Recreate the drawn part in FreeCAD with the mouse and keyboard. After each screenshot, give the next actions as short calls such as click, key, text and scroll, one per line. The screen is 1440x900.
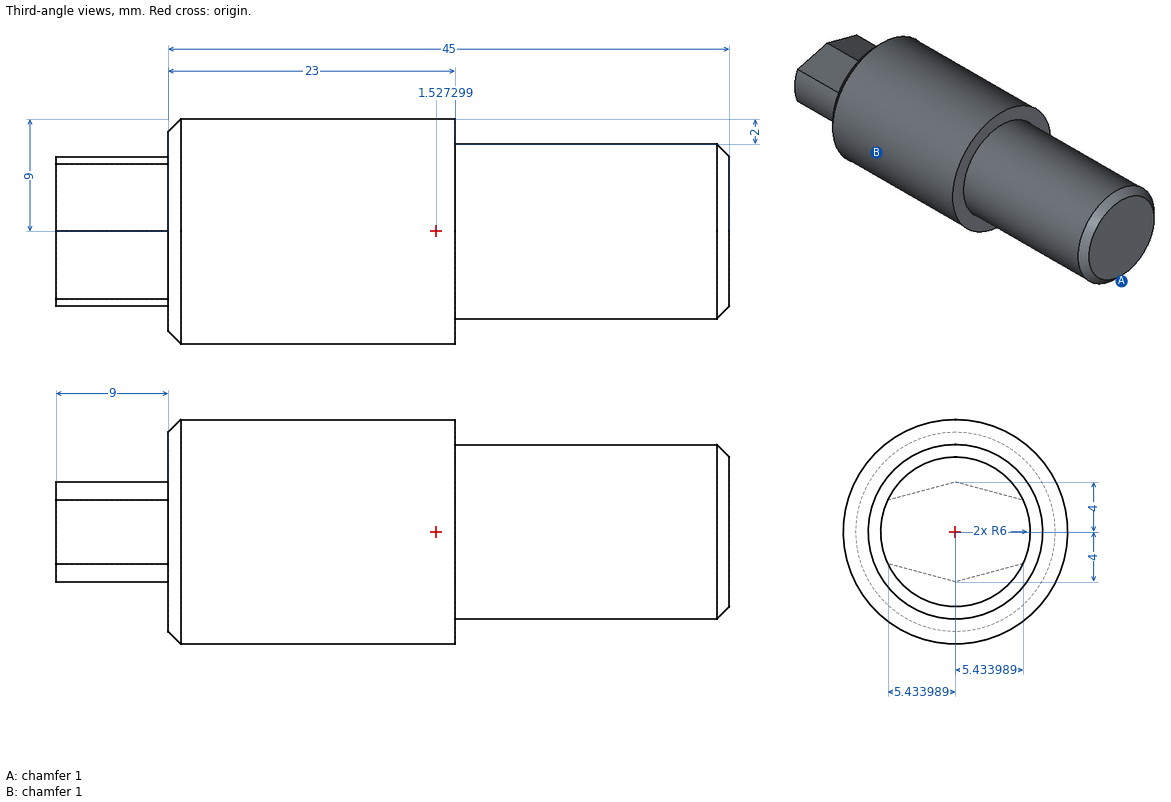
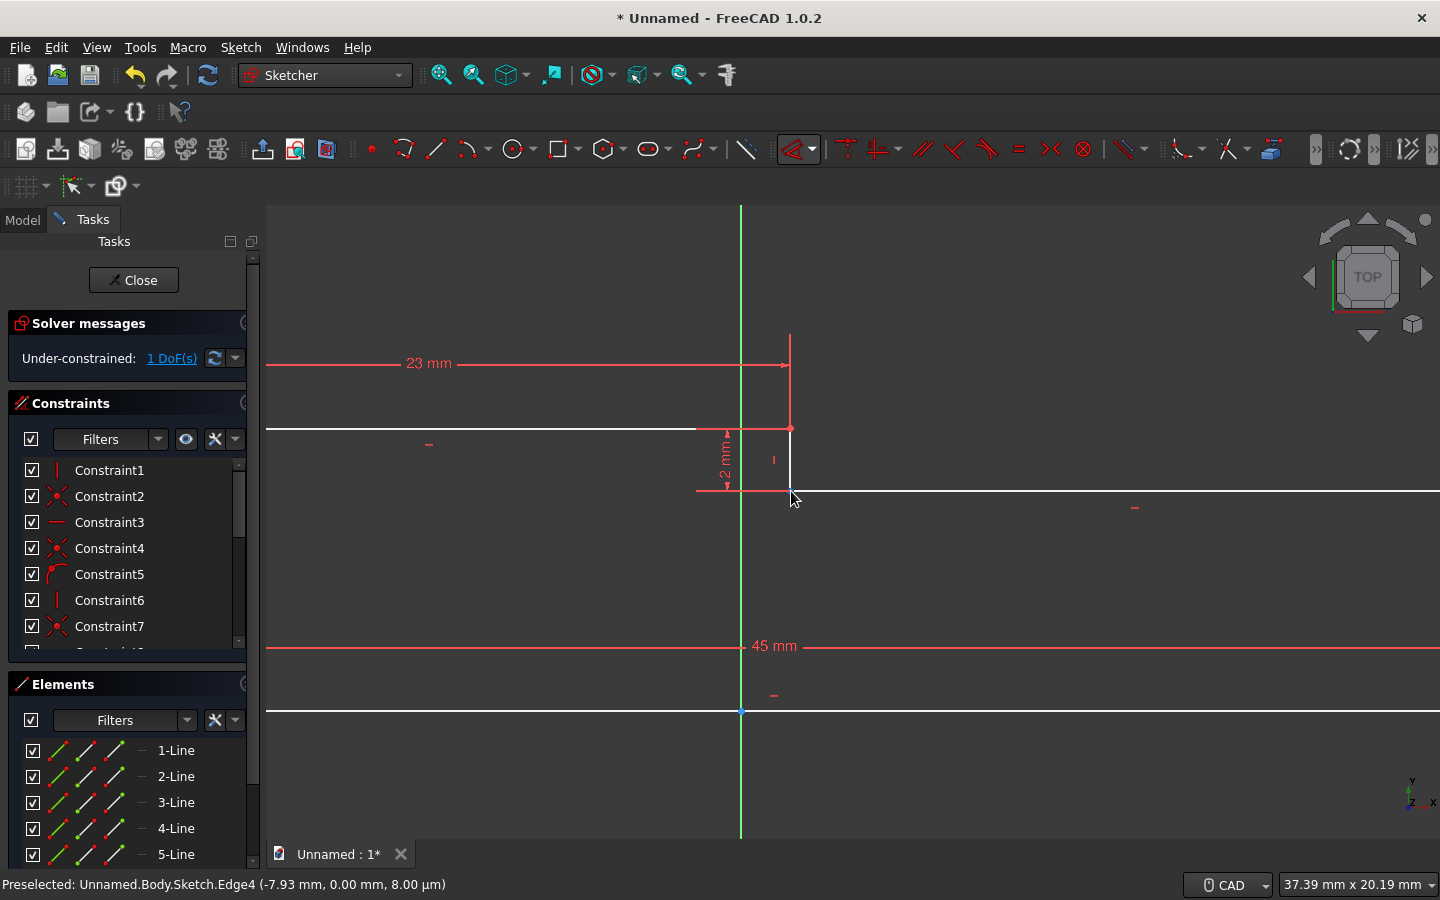
click(790, 491)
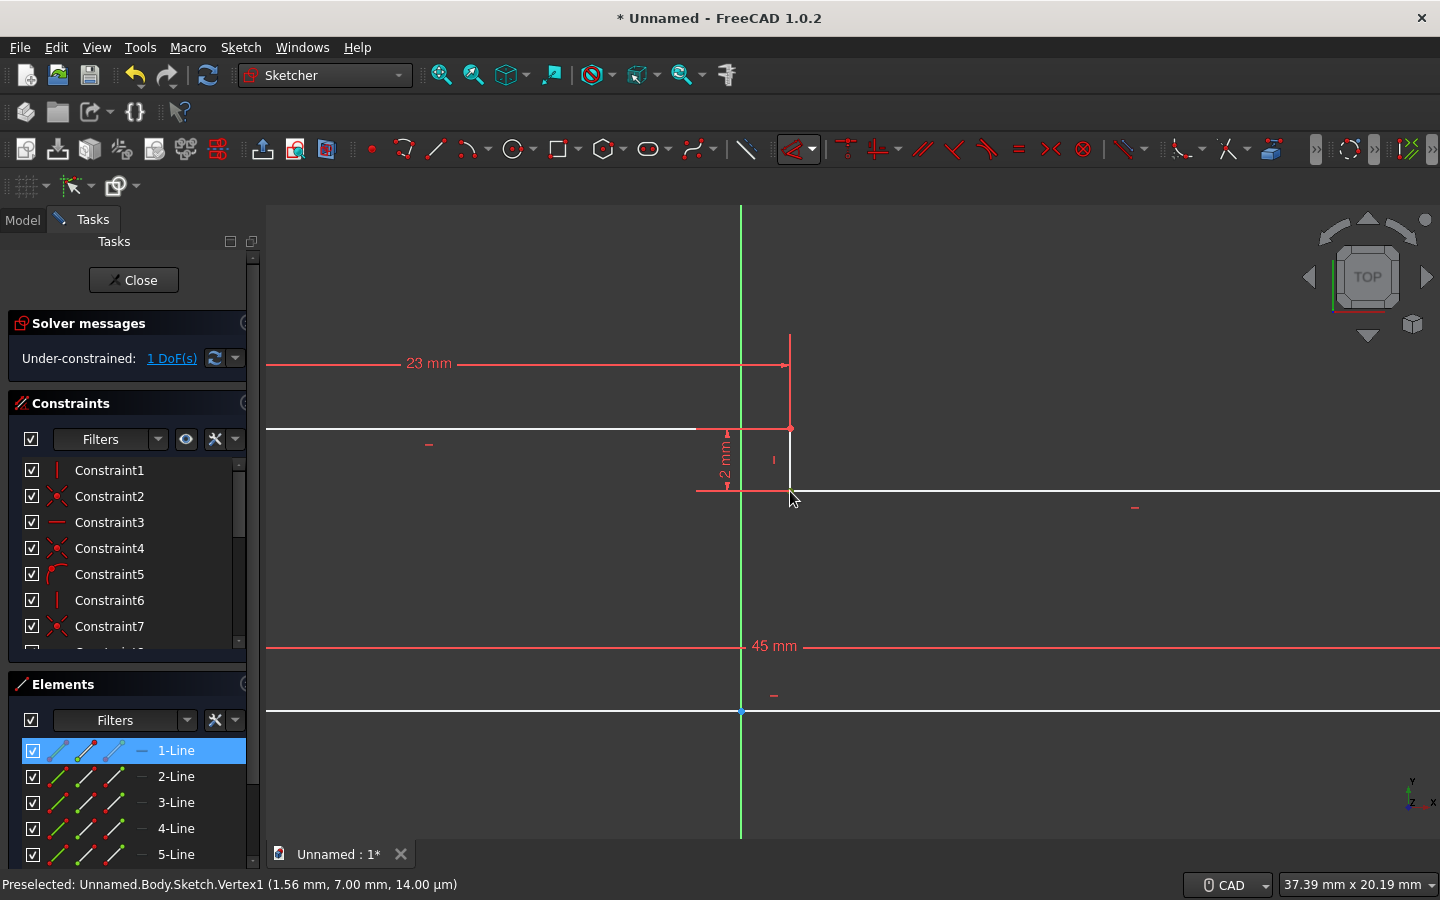
click(814, 150)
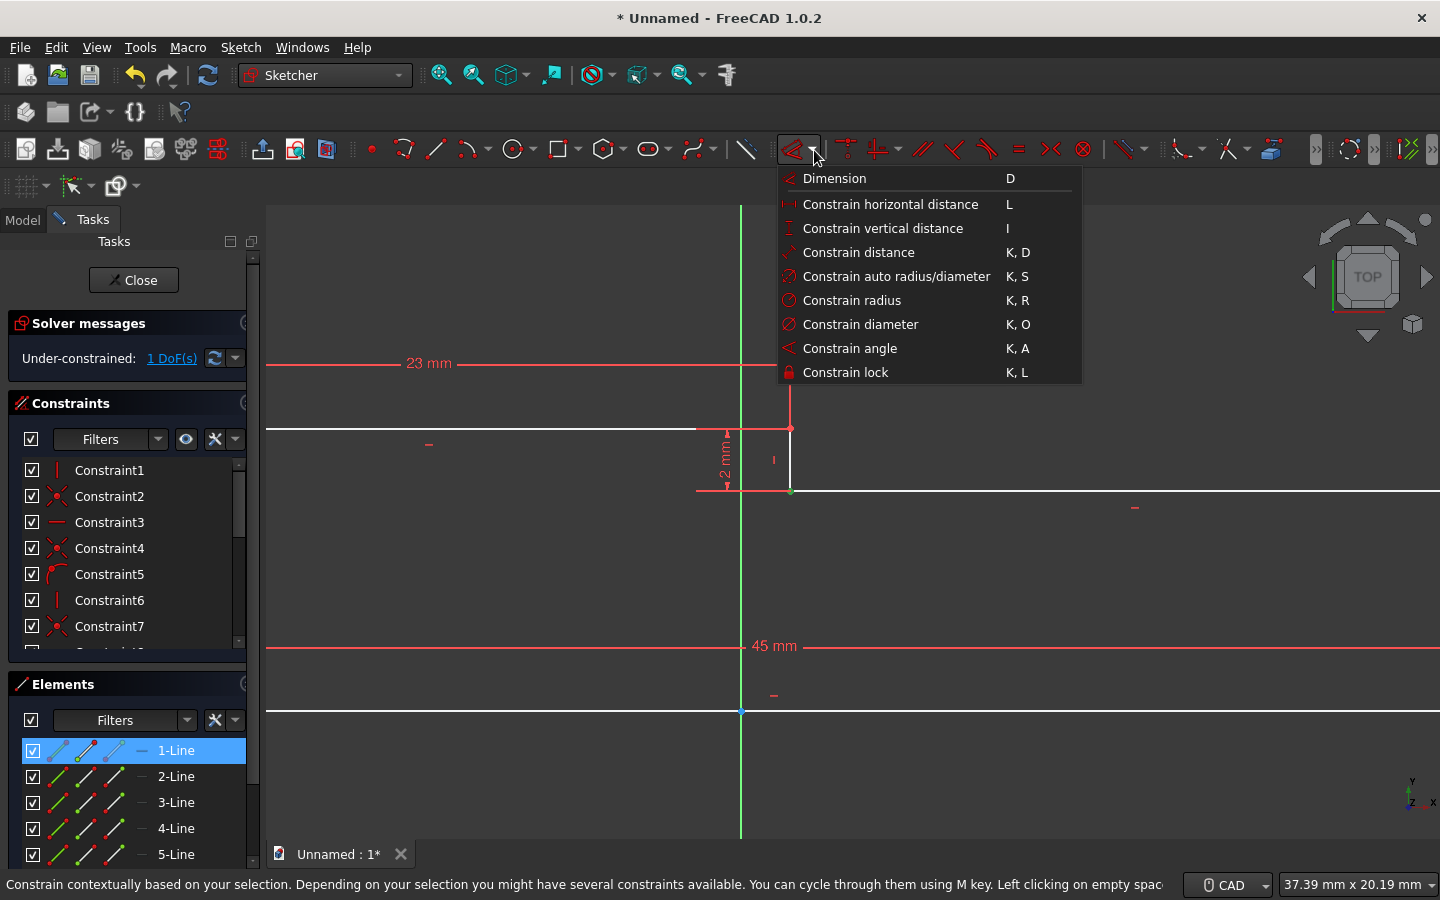
click(930, 204)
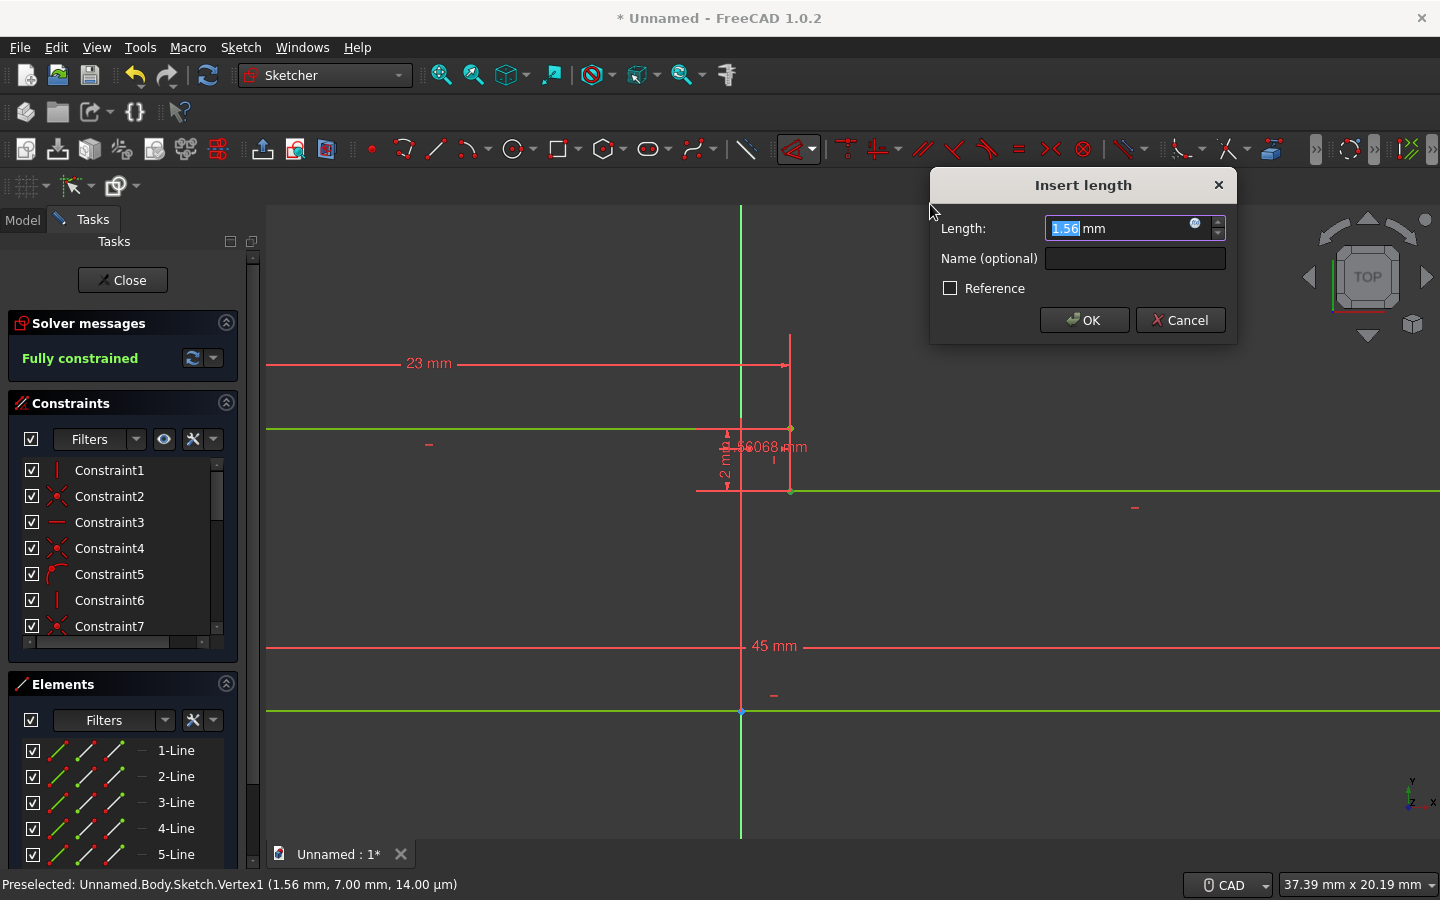
text(1.527299)
key(Return)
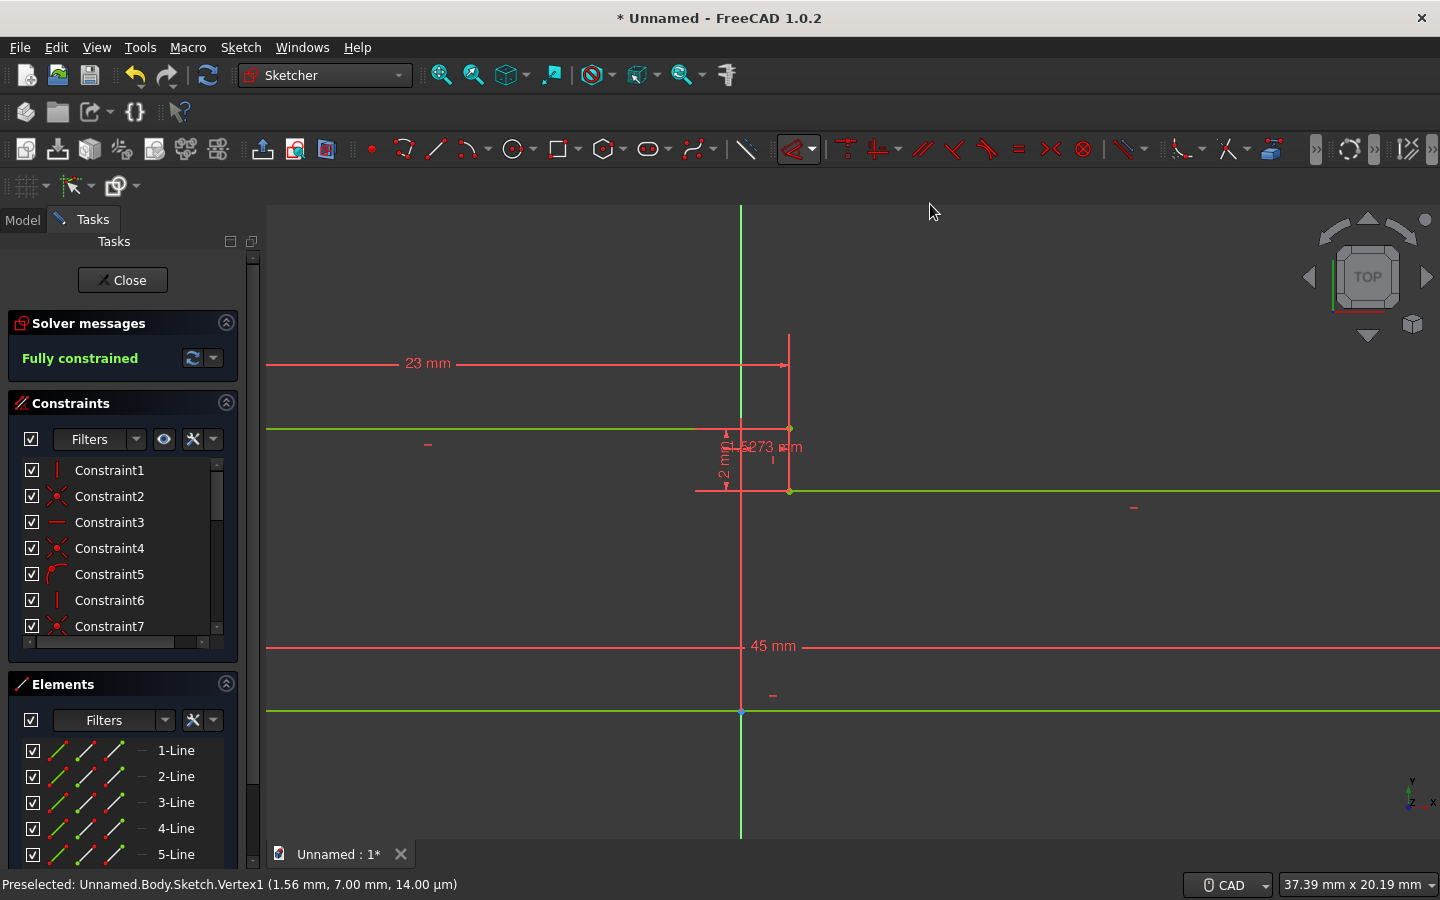
click(123, 280)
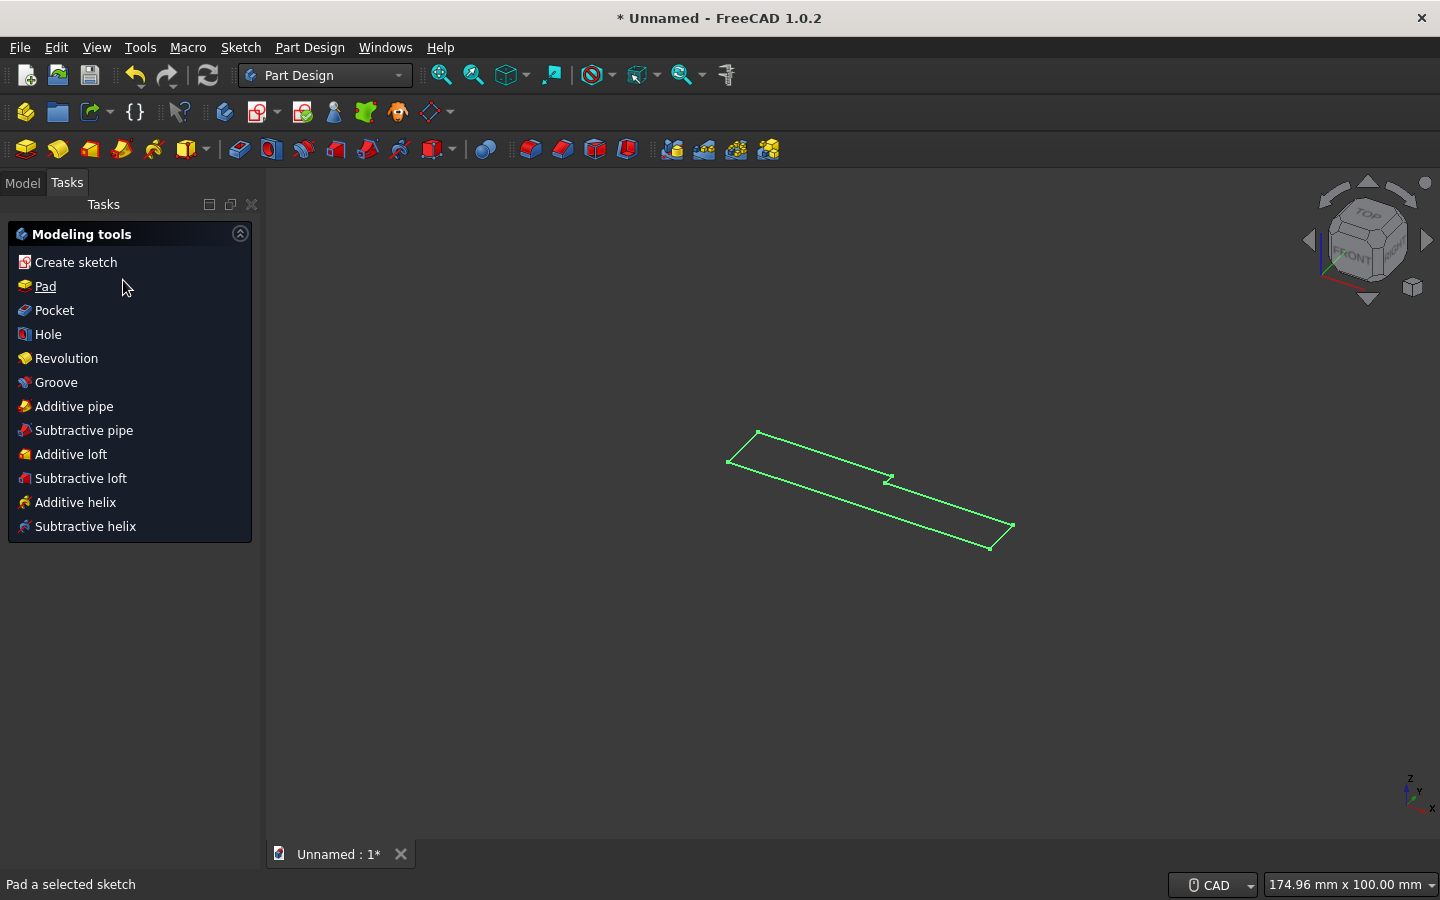
click(58, 150)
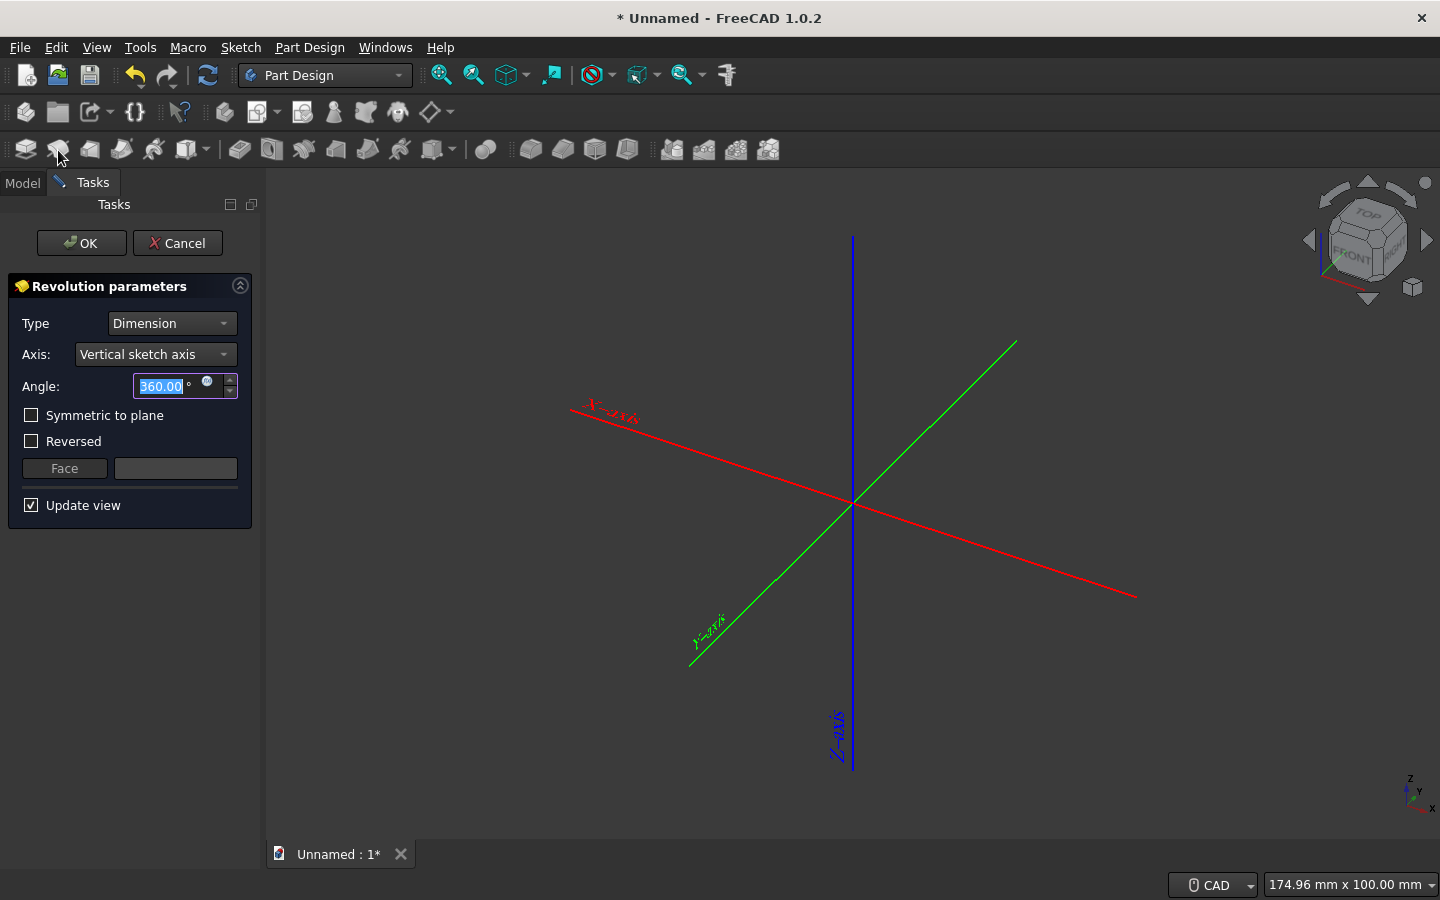
click(156, 354)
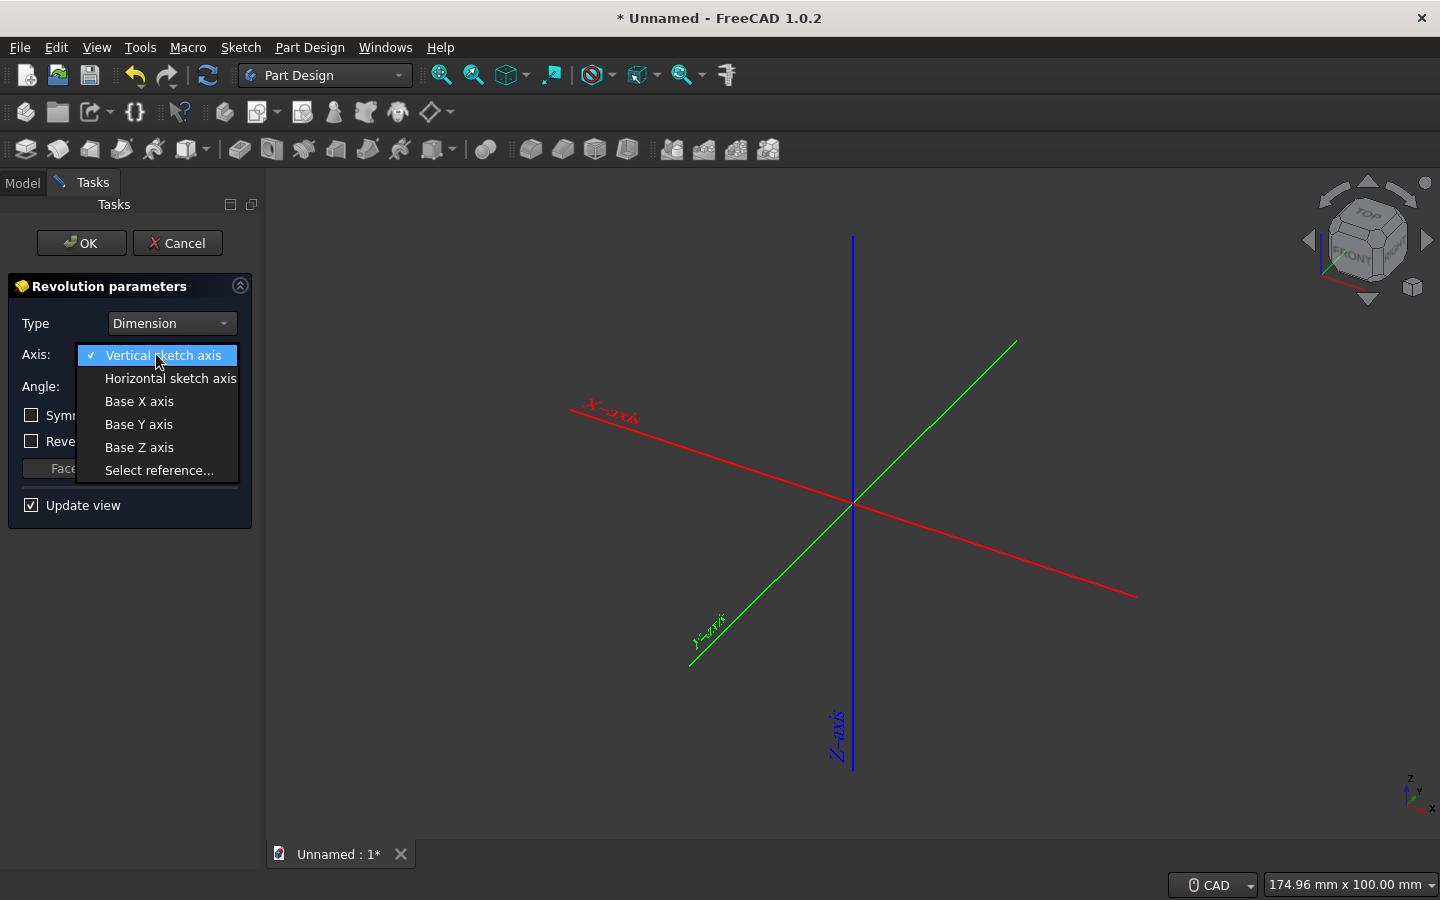
click(156, 378)